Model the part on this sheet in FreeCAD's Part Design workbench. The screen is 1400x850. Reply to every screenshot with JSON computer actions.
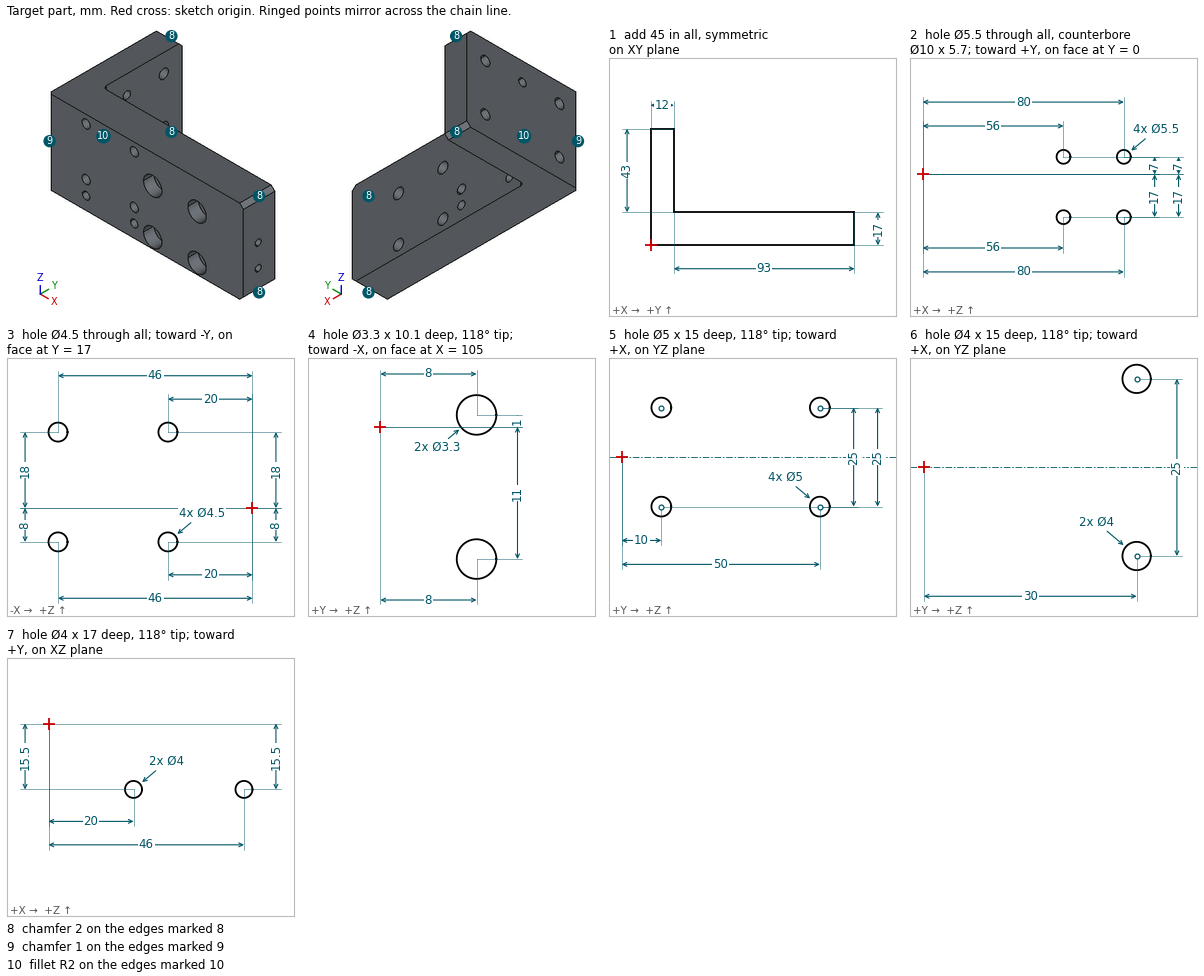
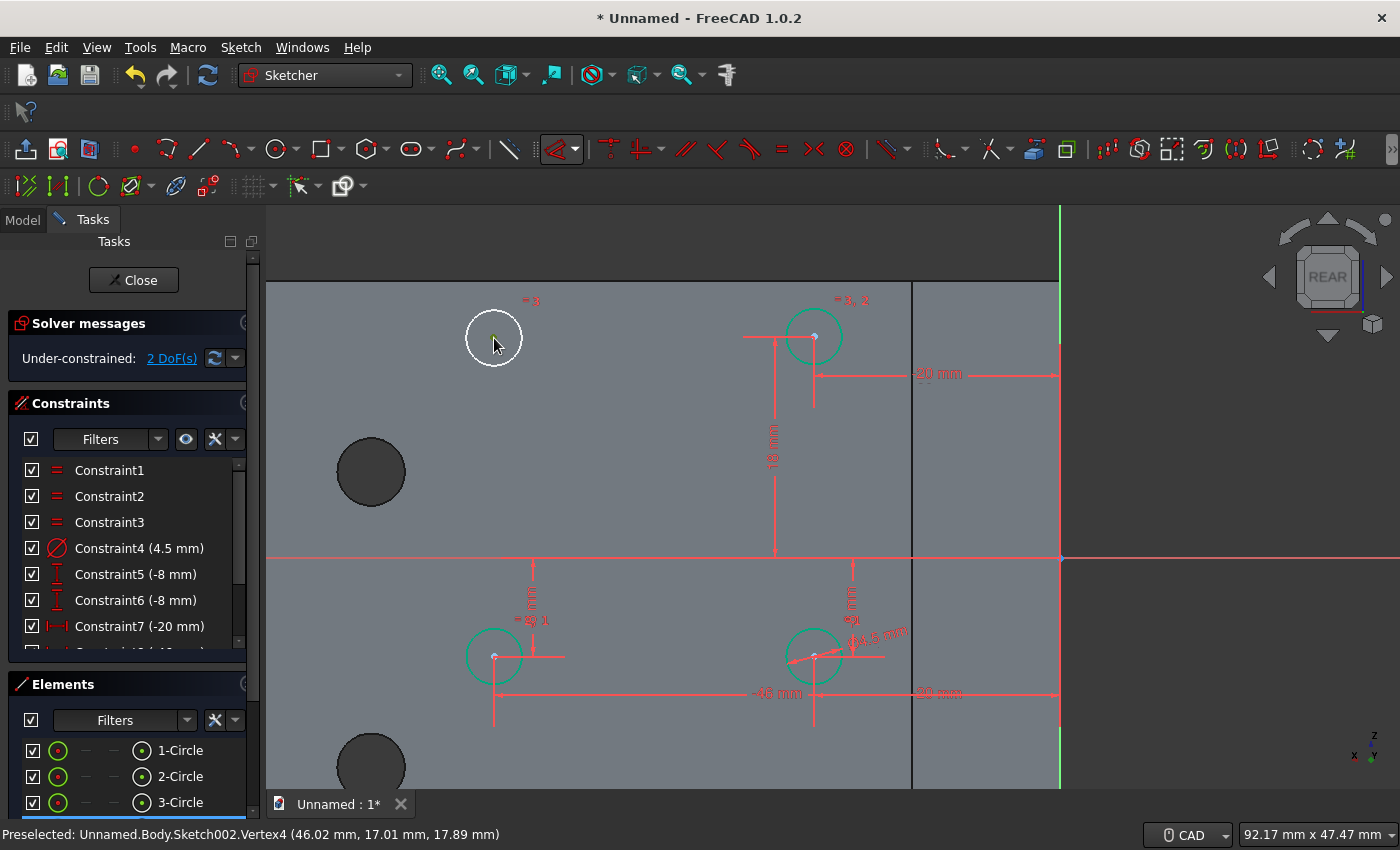
{"action": "key", "text": "l"}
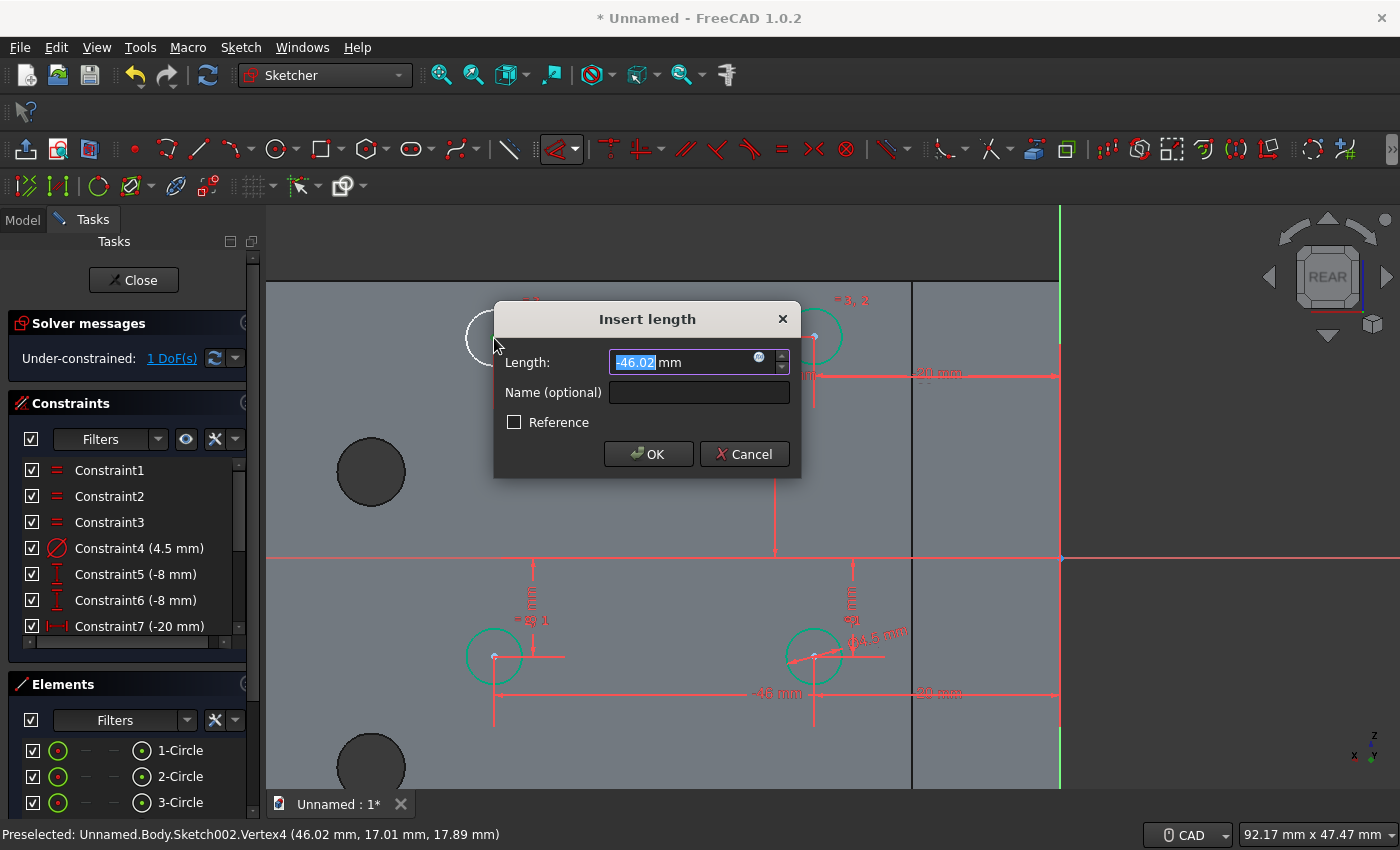
{"action": "type", "text": "-46"}
{"action": "key", "text": "Return"}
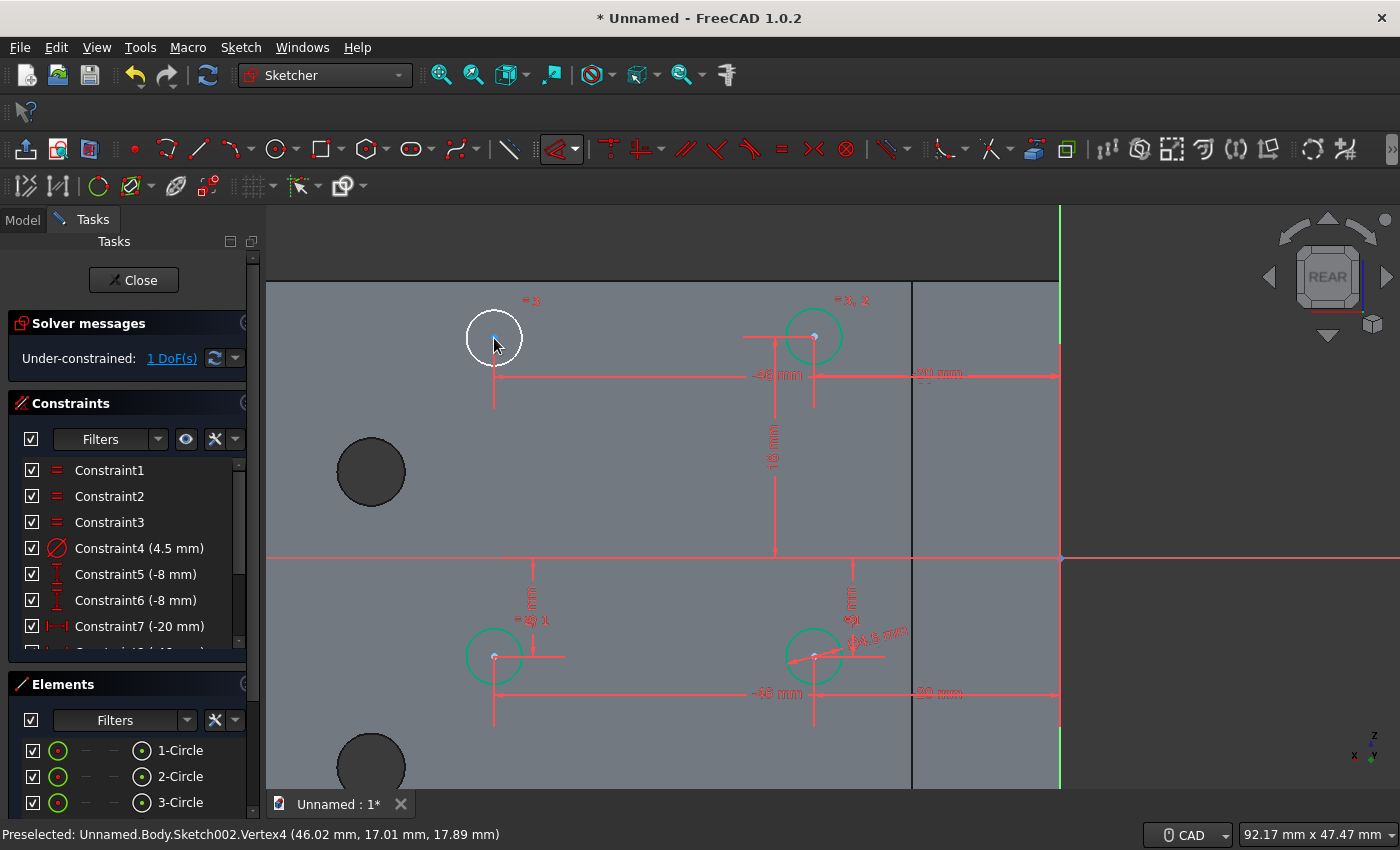
{"action": "left_click", "coordinate": [494, 338]}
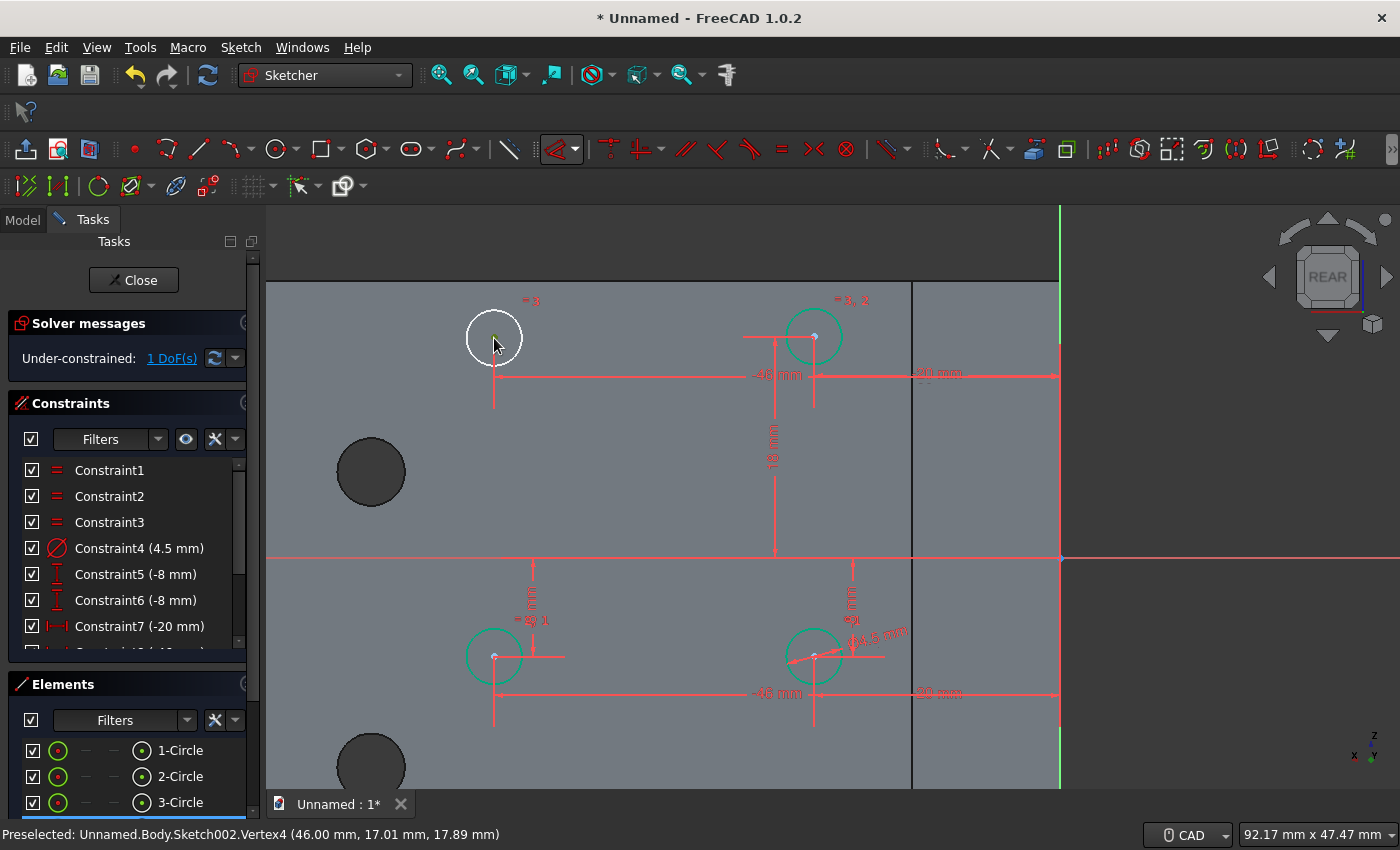
{"action": "key", "text": "i"}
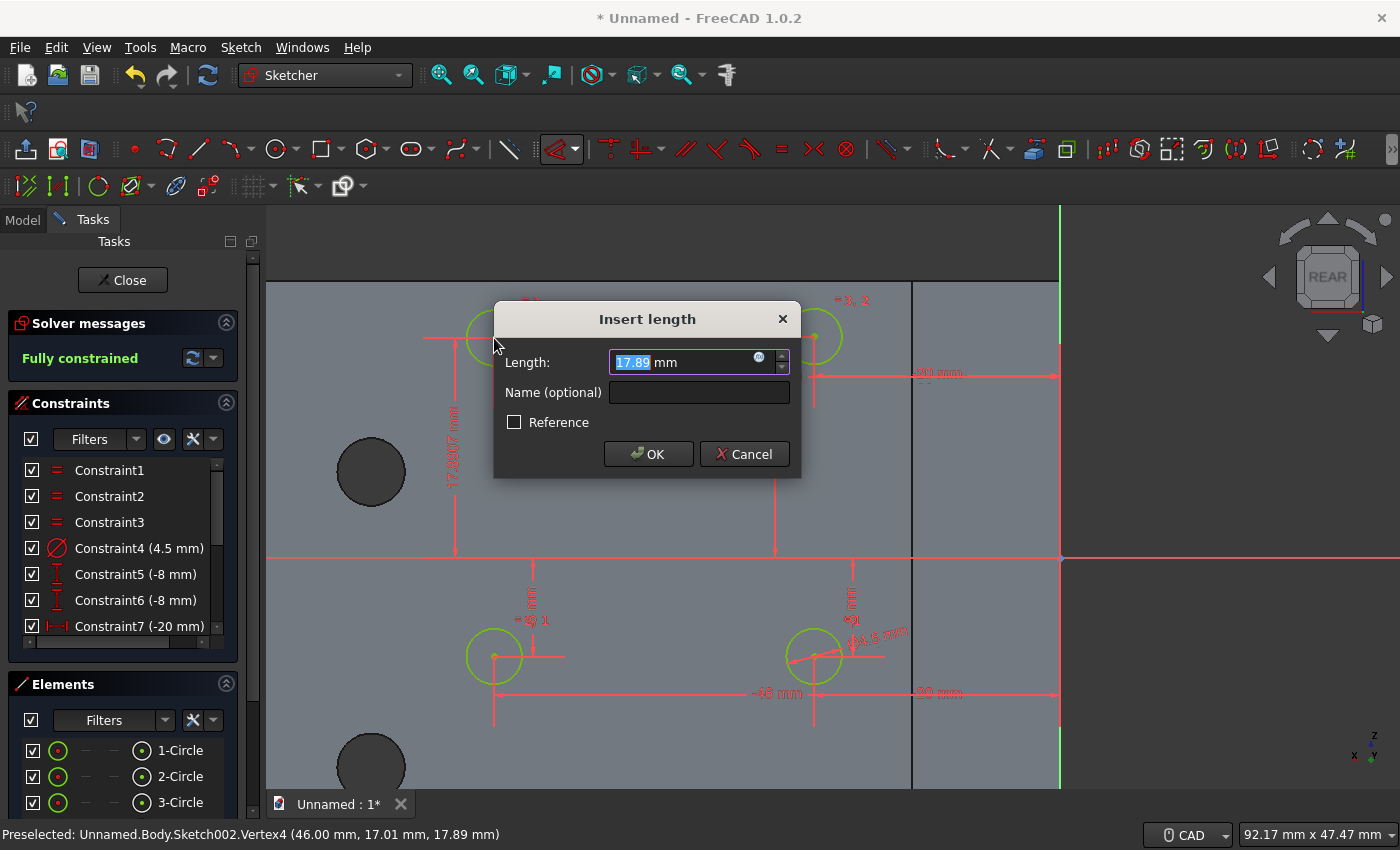
{"action": "type", "text": "18"}
{"action": "key", "text": "Return"}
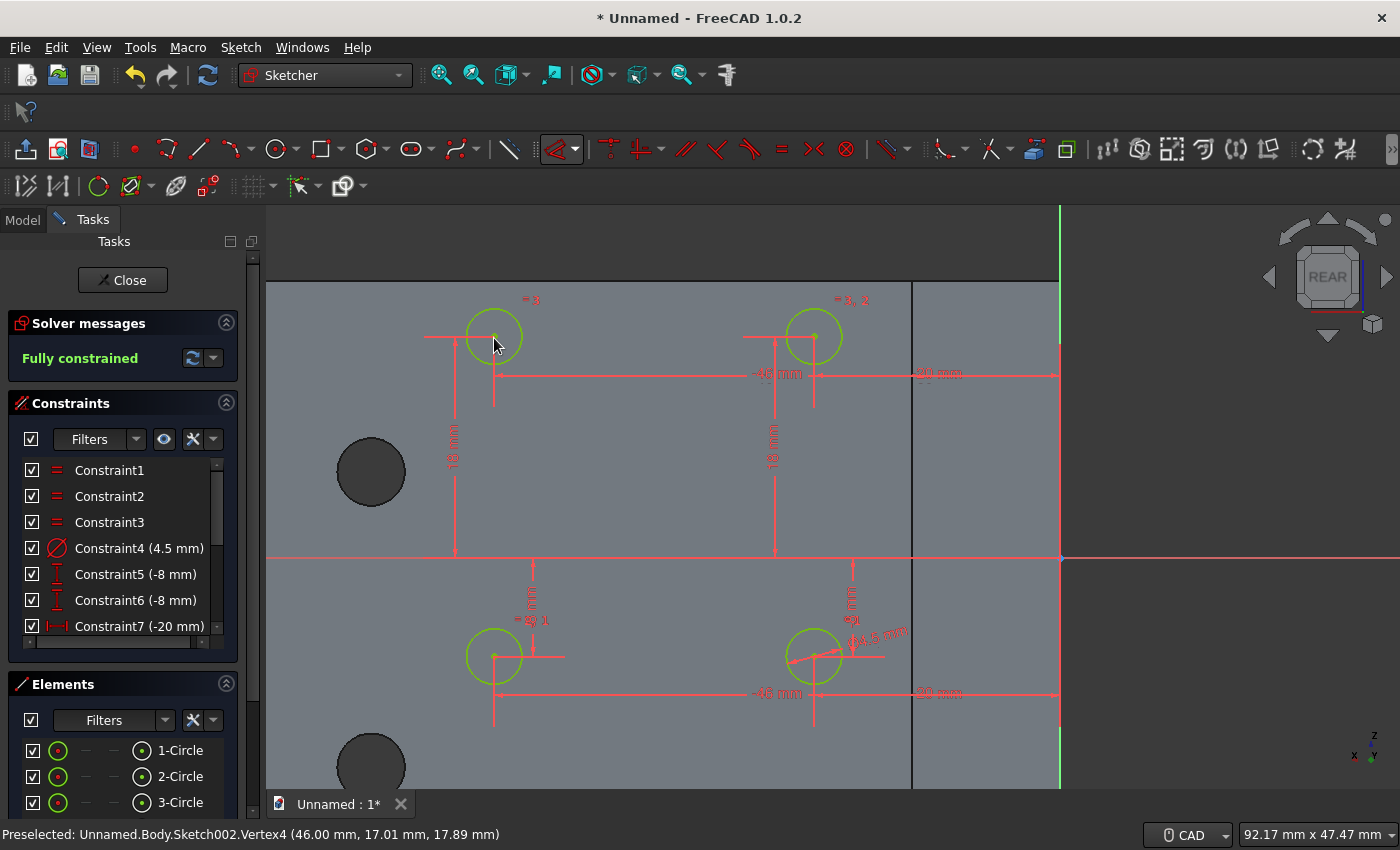
{"action": "left_click", "coordinate": [123, 280]}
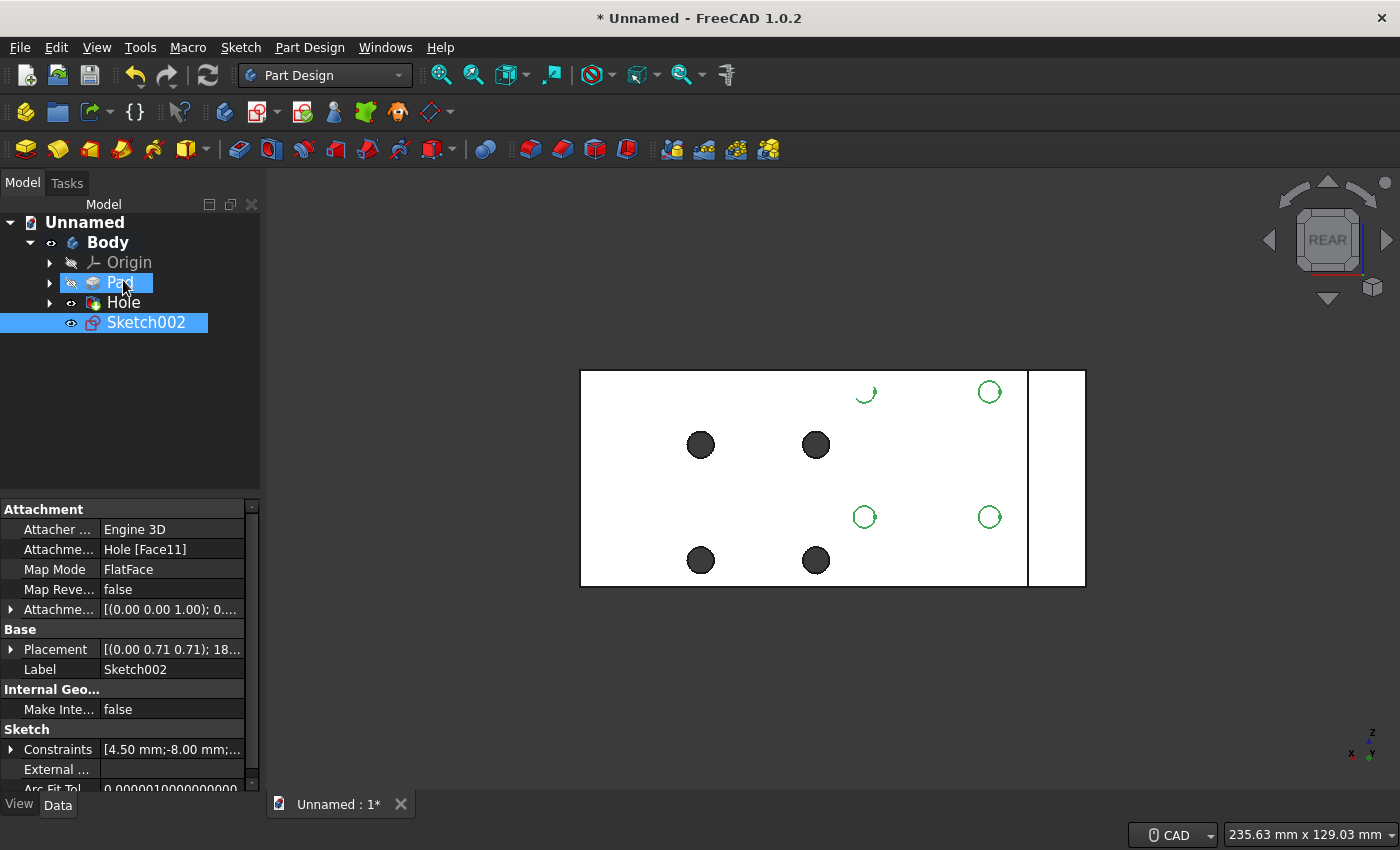
{"action": "left_click", "coordinate": [272, 150]}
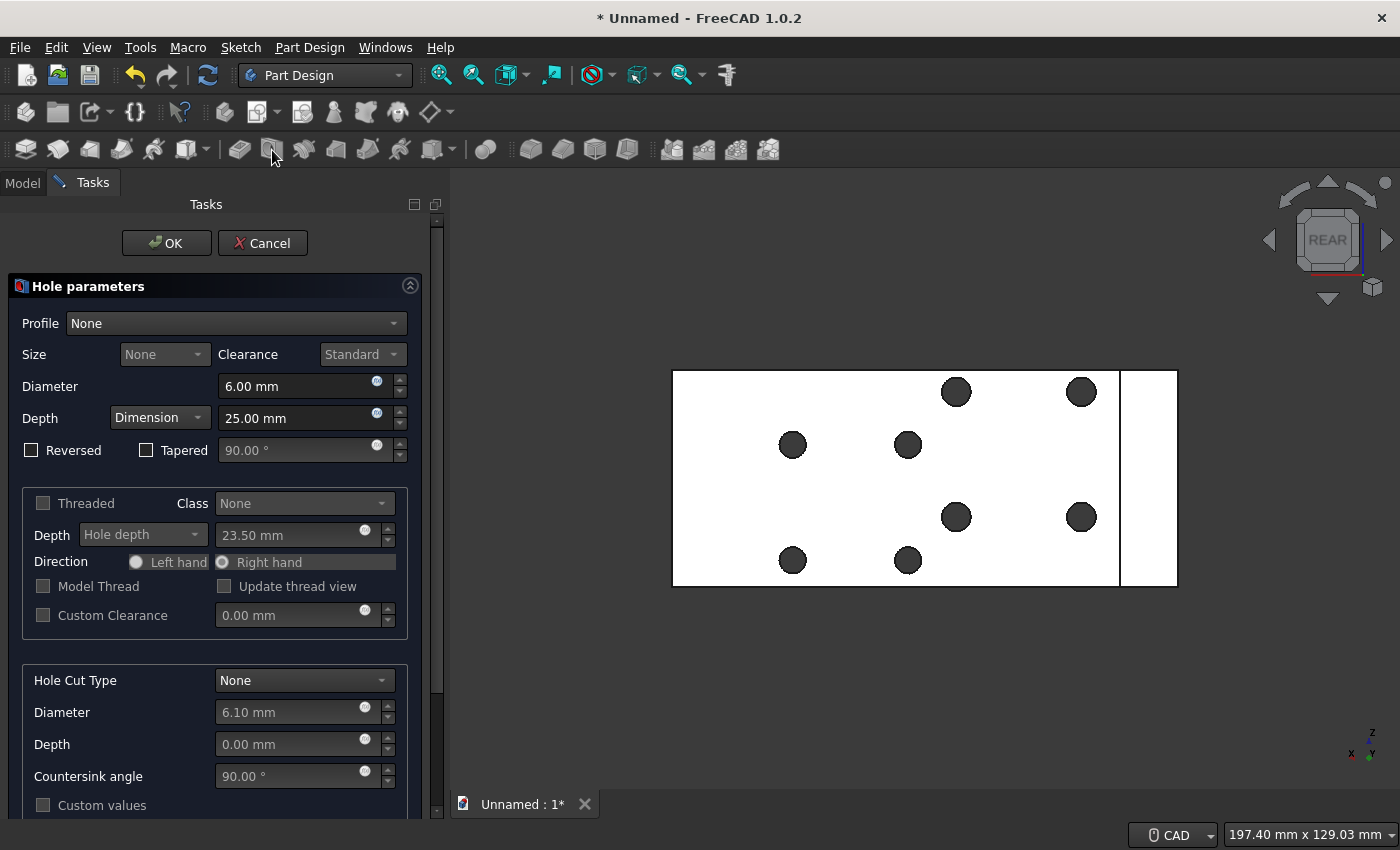
{"action": "triple_click", "coordinate": [305, 386]}